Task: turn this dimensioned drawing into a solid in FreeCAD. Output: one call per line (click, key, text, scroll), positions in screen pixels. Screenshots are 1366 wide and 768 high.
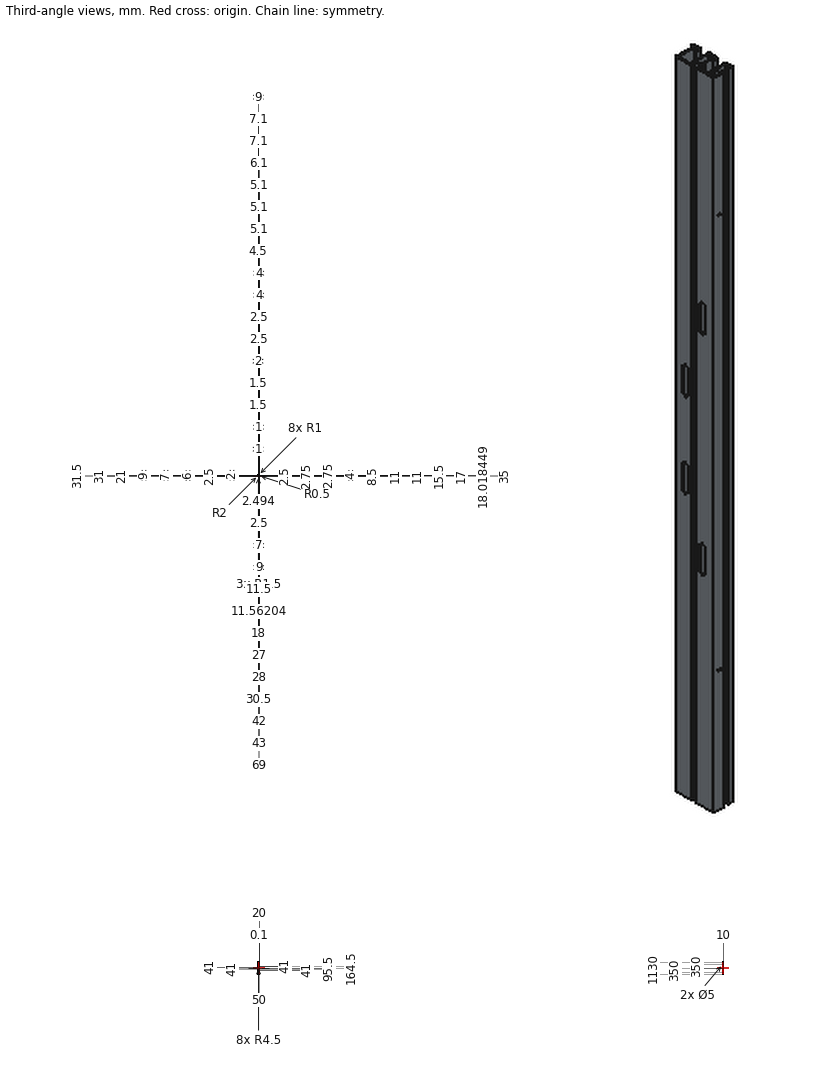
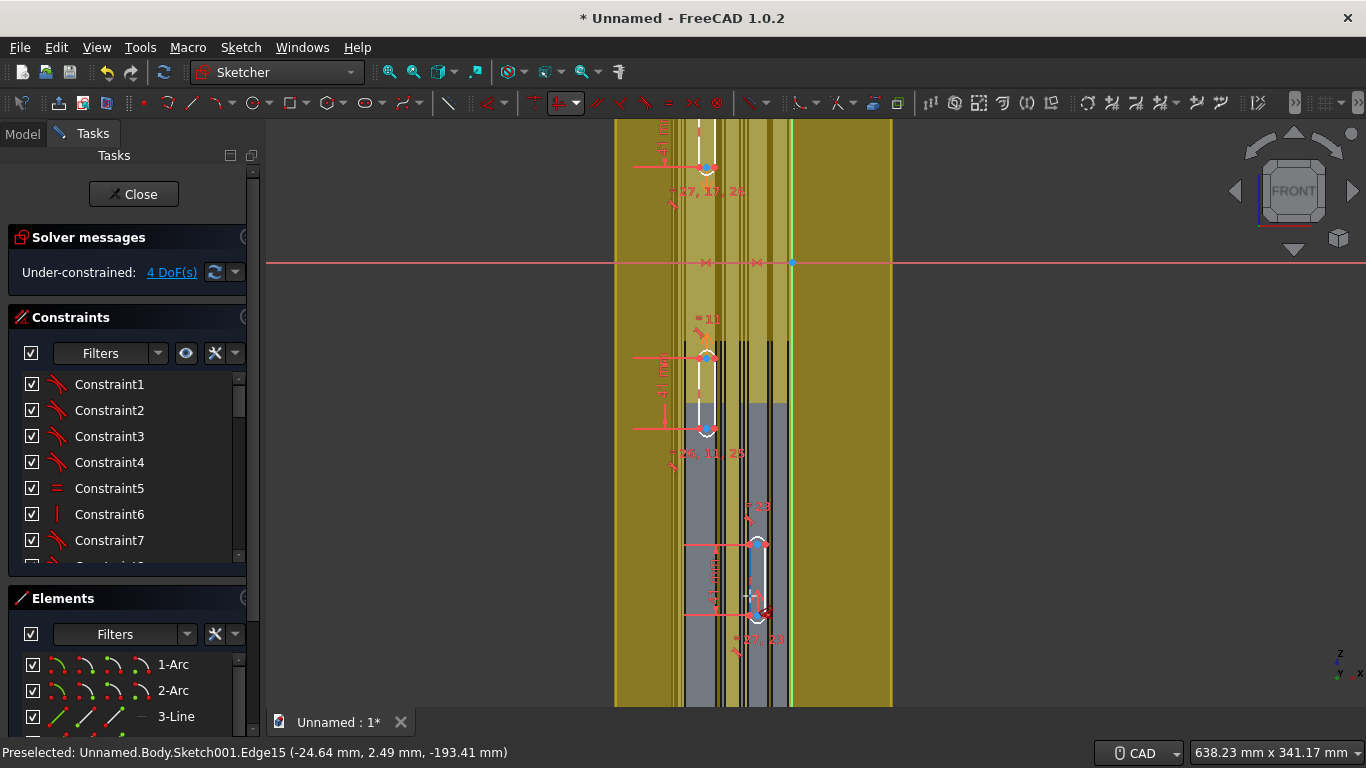
scroll(754, 259, up, 6)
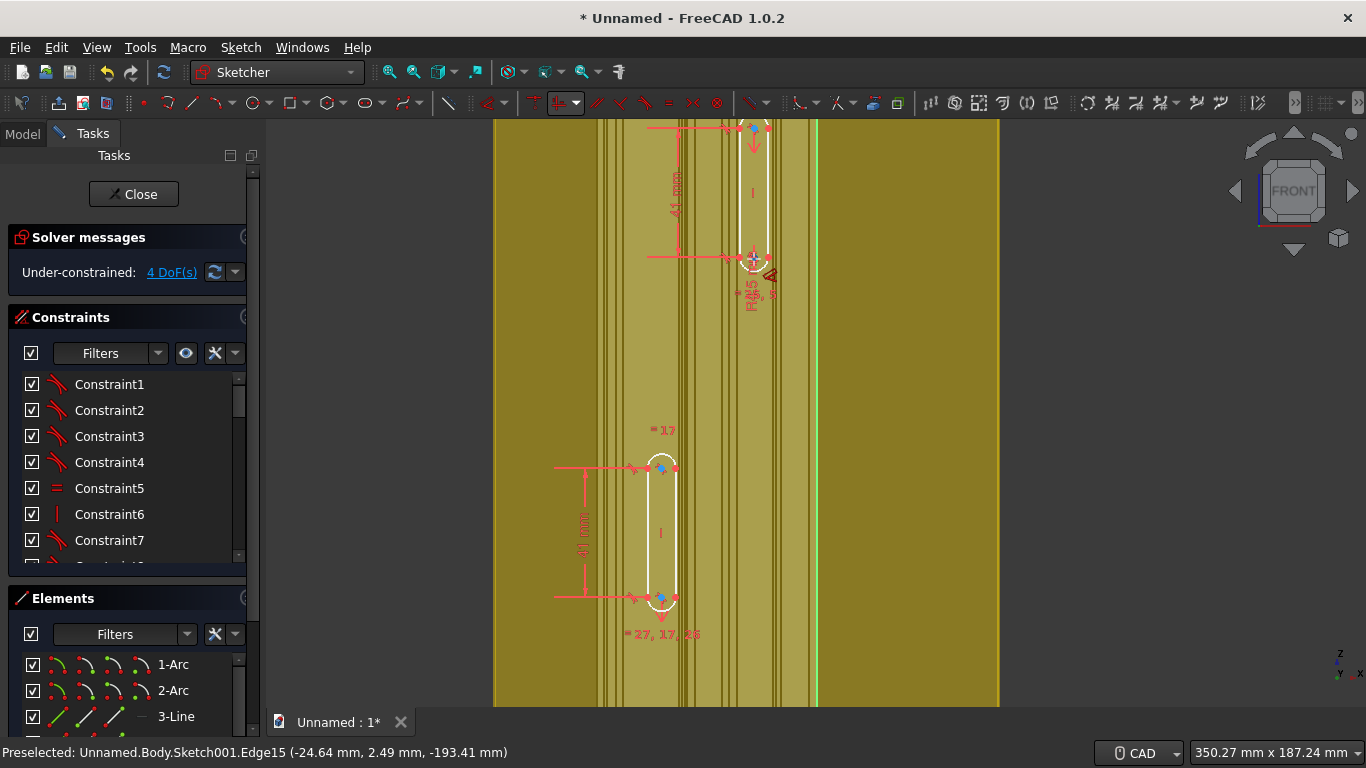
click(754, 257)
click(786, 223)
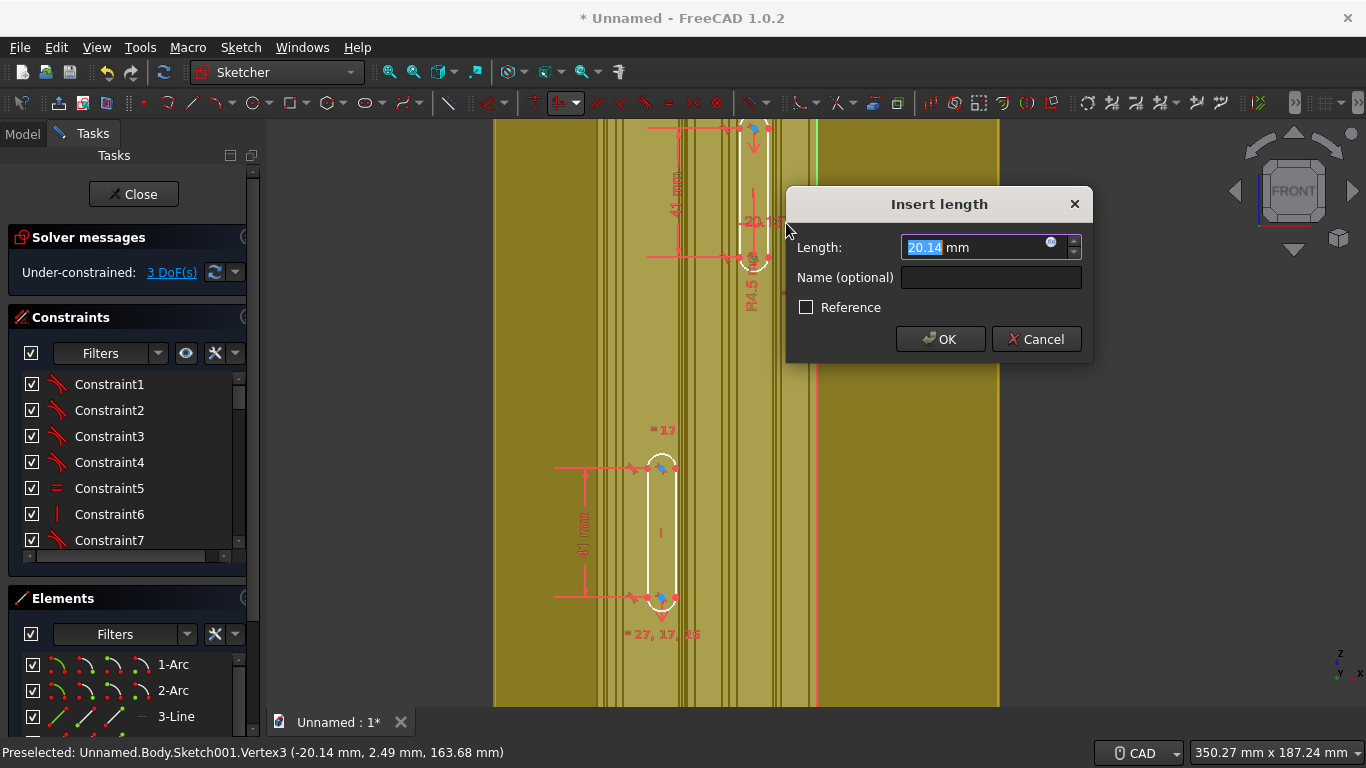
text(20)
key(Return)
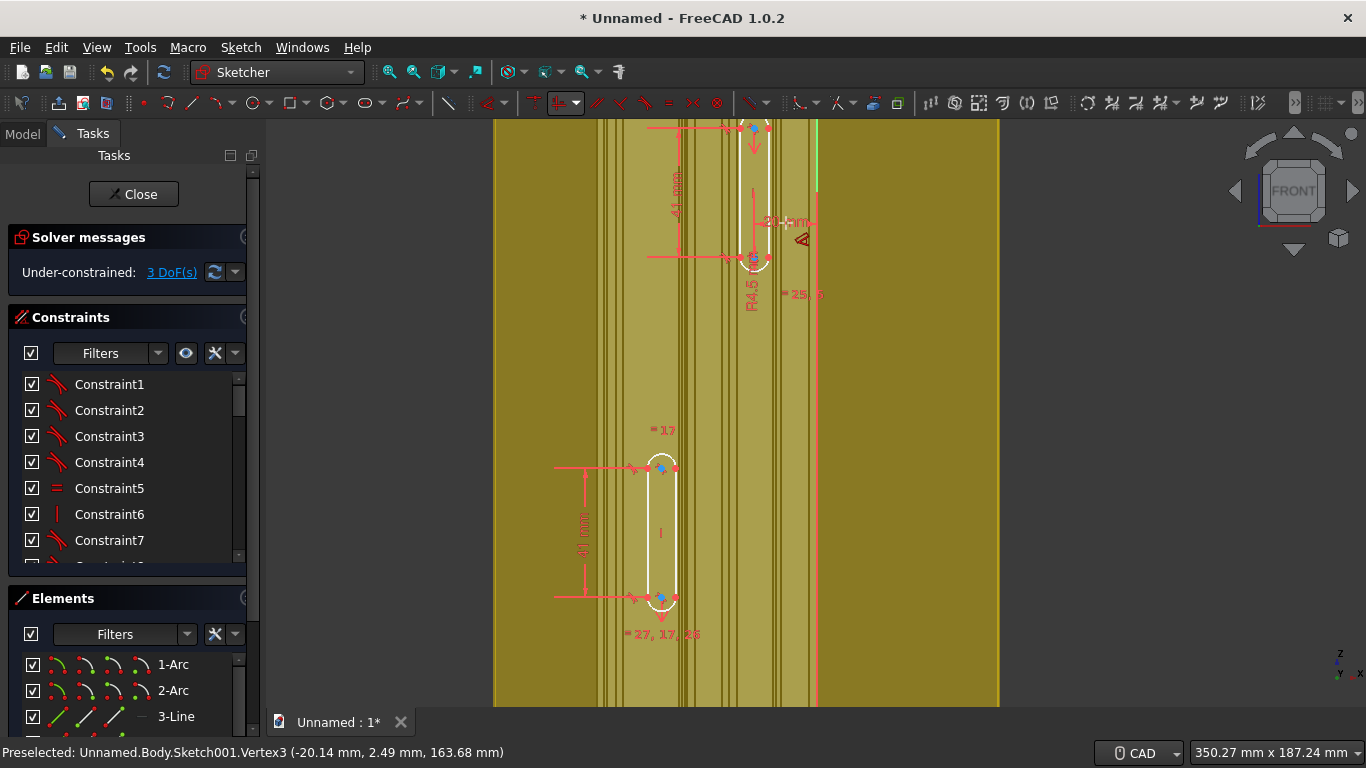
scroll(754, 259, down, 6)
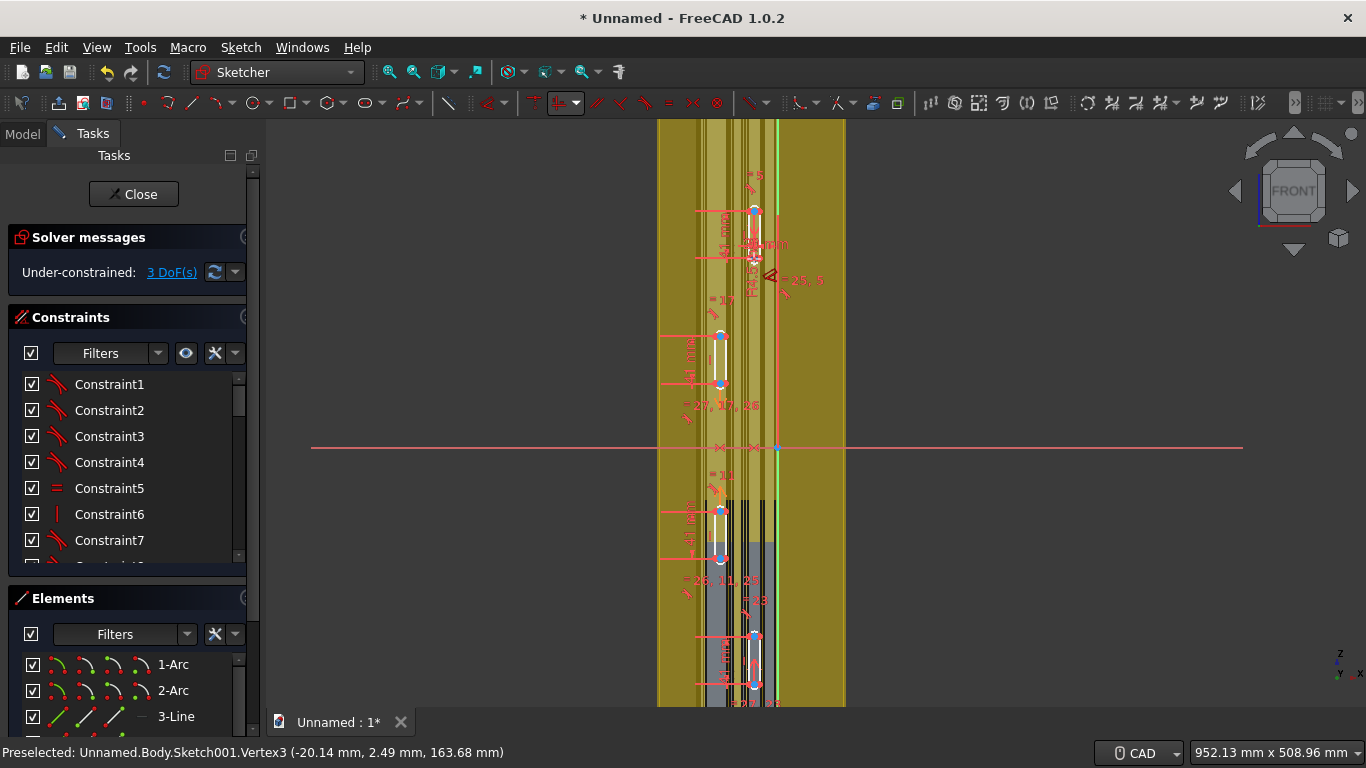
scroll(727, 505, up, 6)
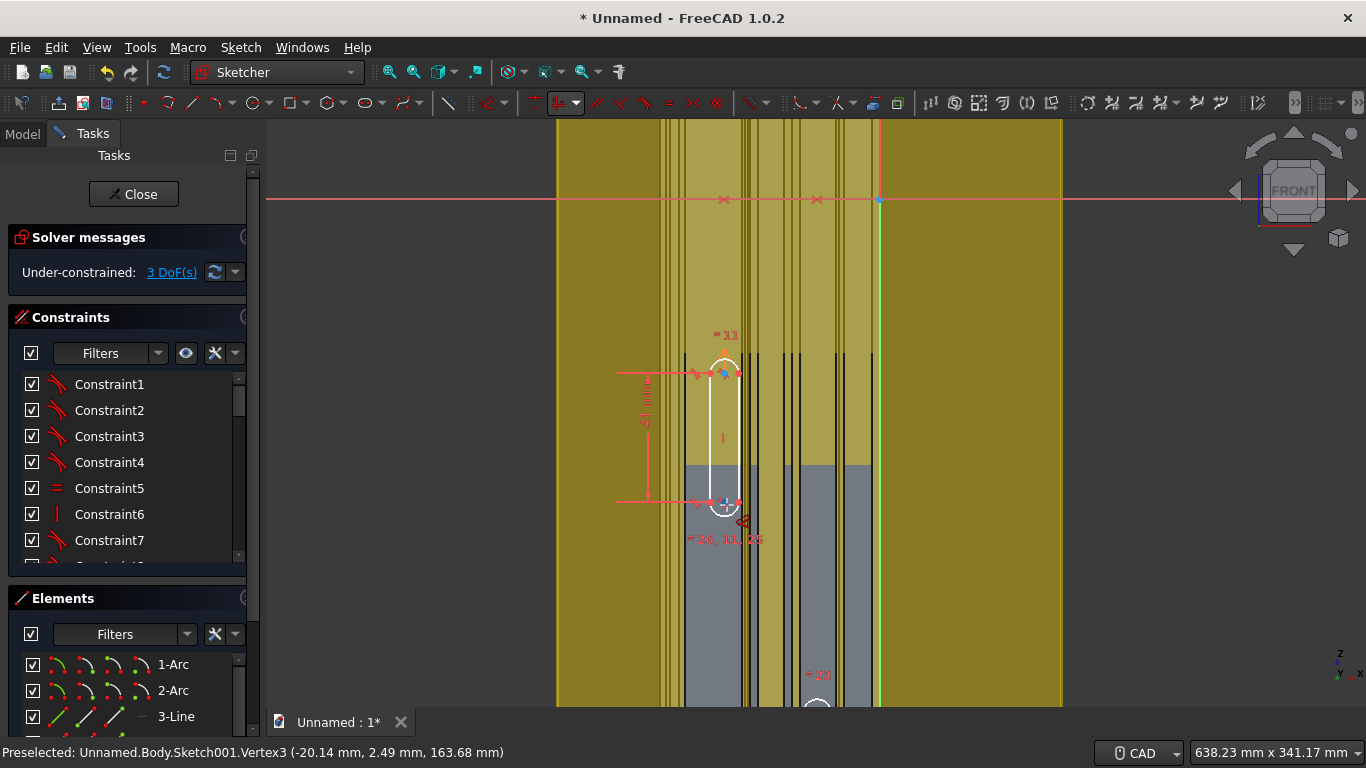
click(725, 502)
click(802, 536)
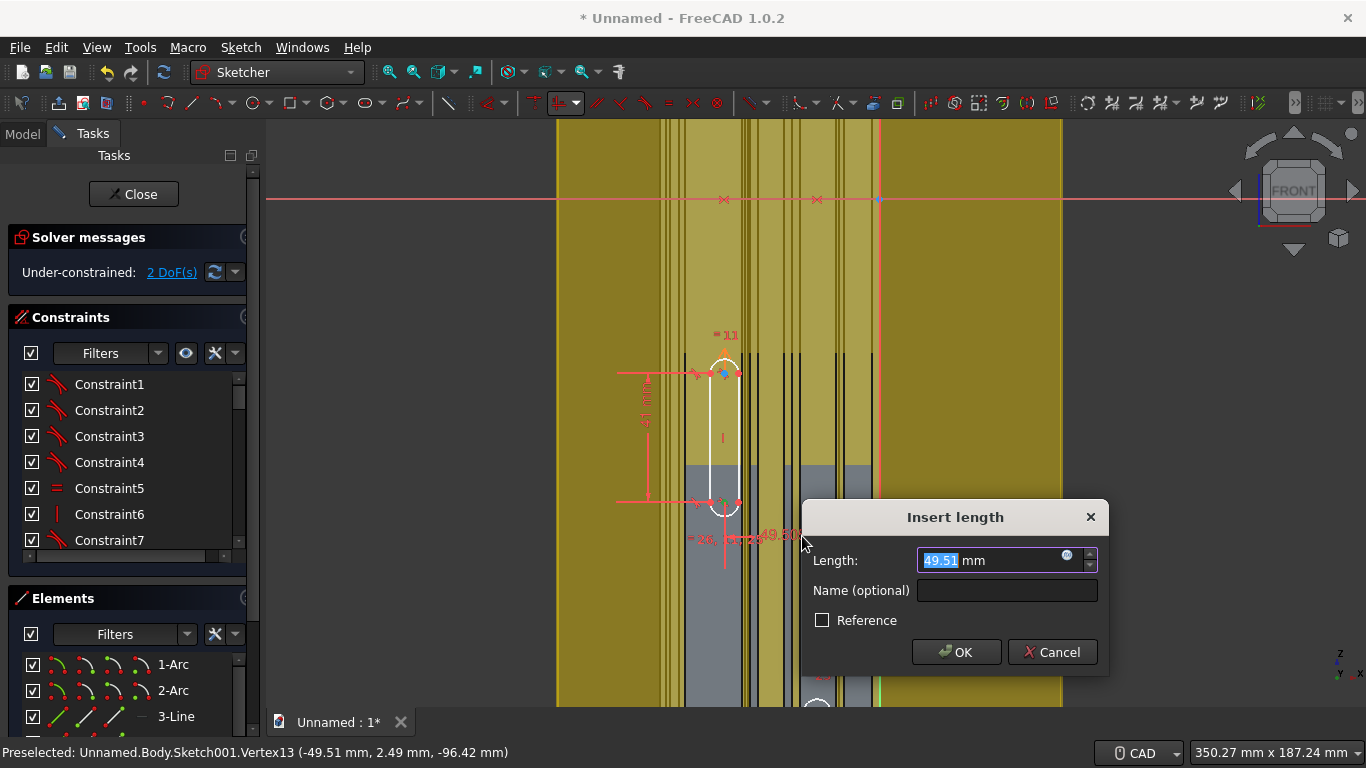
text(50)
key(Return)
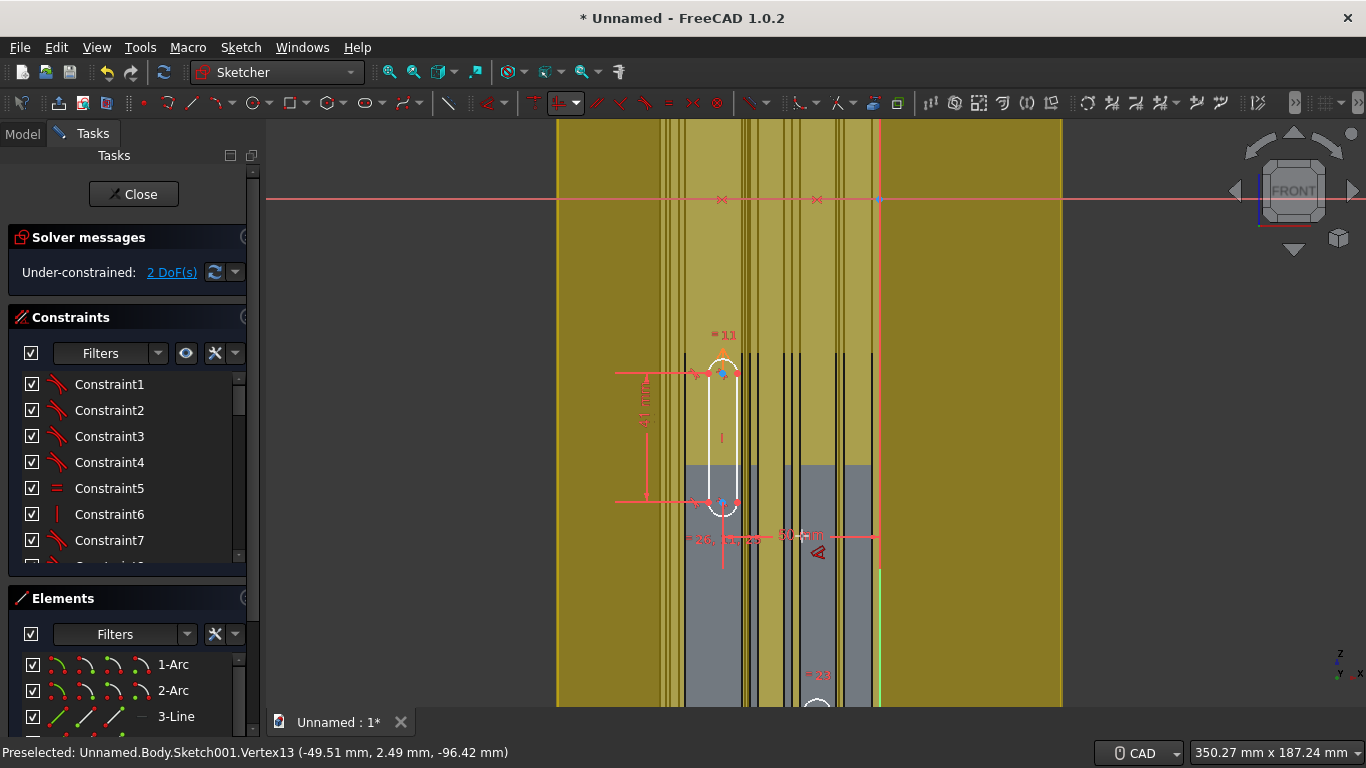
click(709, 502)
click(914, 351)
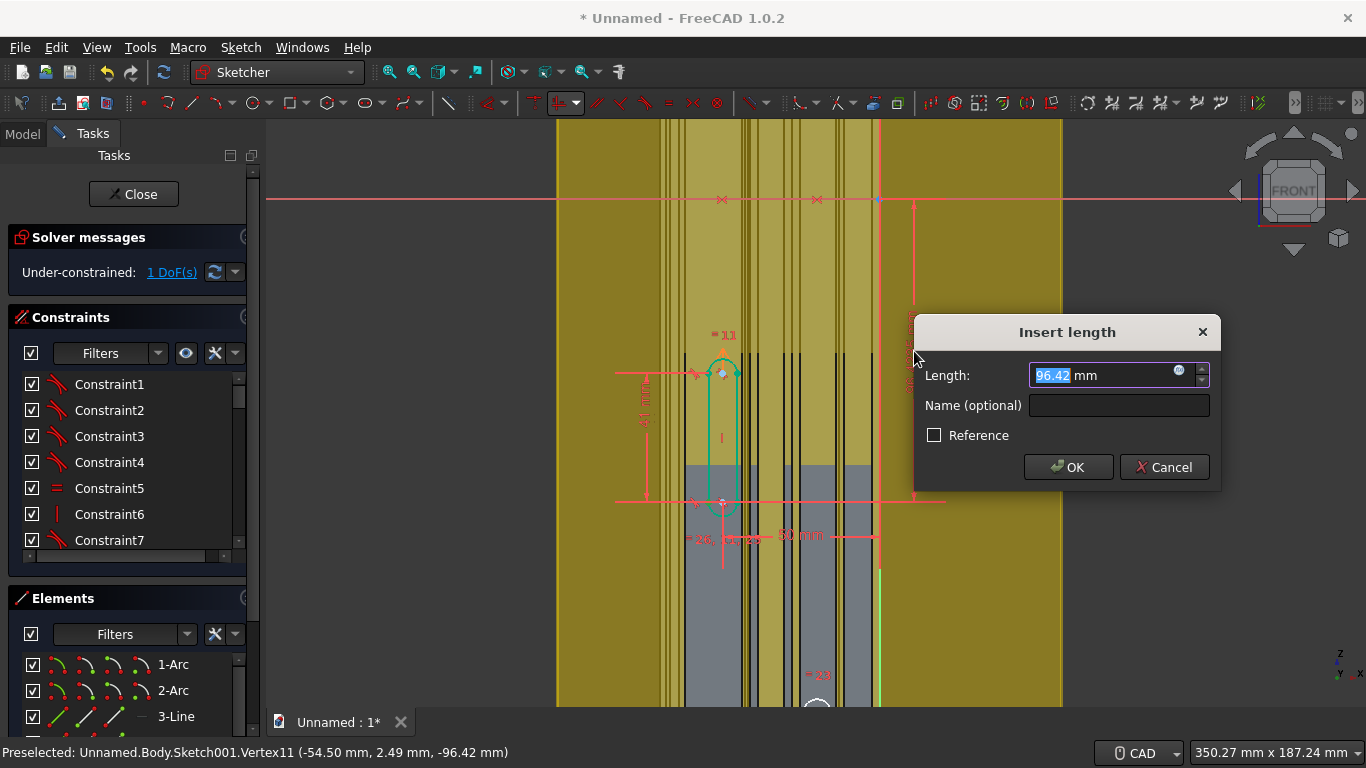
text(95.5)
key(Return)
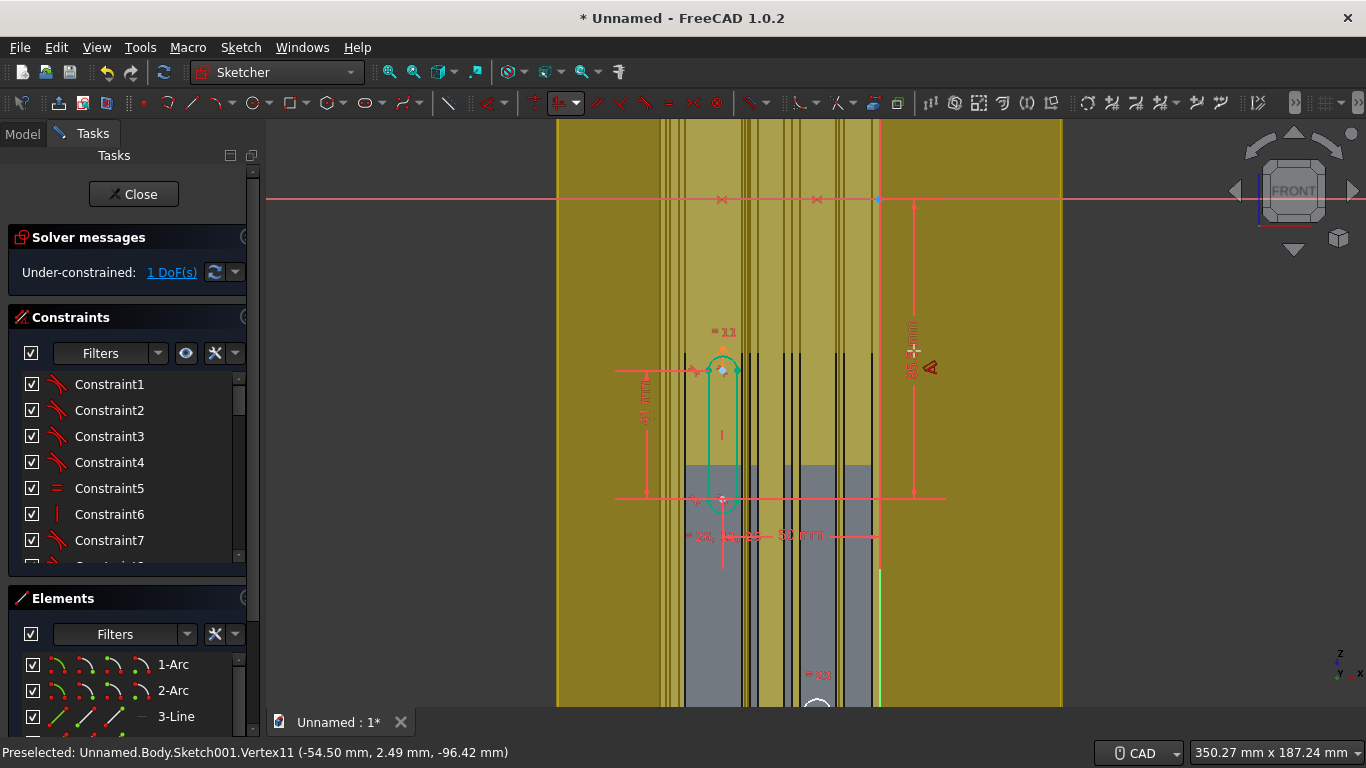
scroll(727, 505, down, 6)